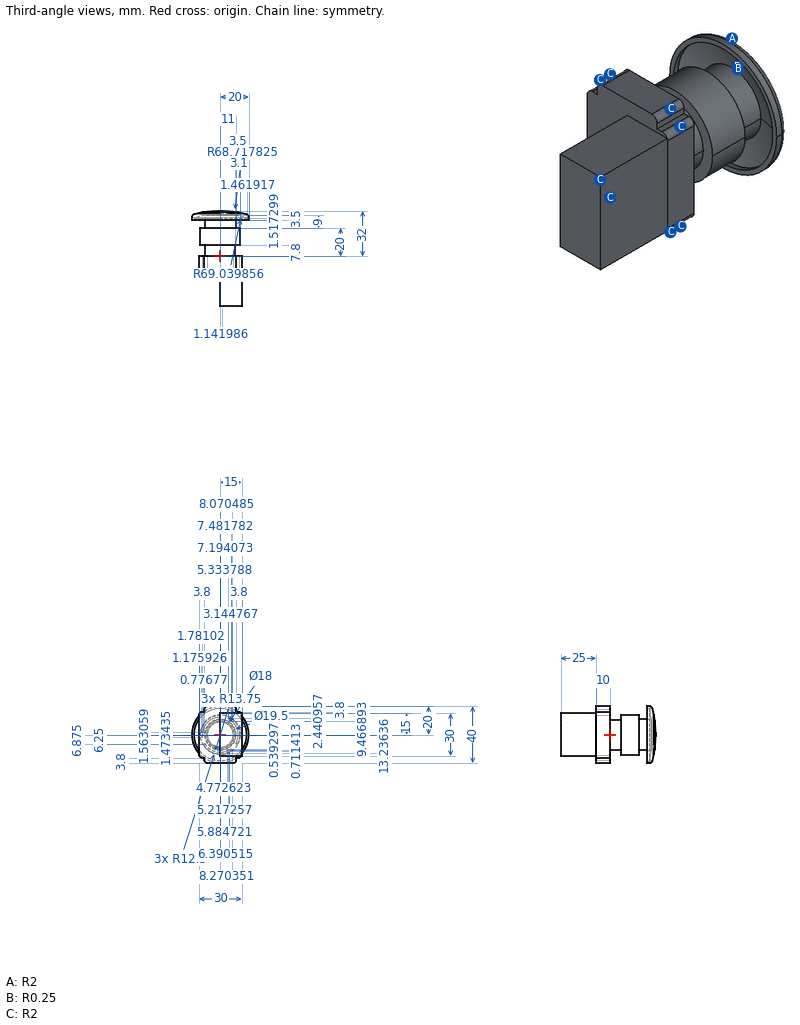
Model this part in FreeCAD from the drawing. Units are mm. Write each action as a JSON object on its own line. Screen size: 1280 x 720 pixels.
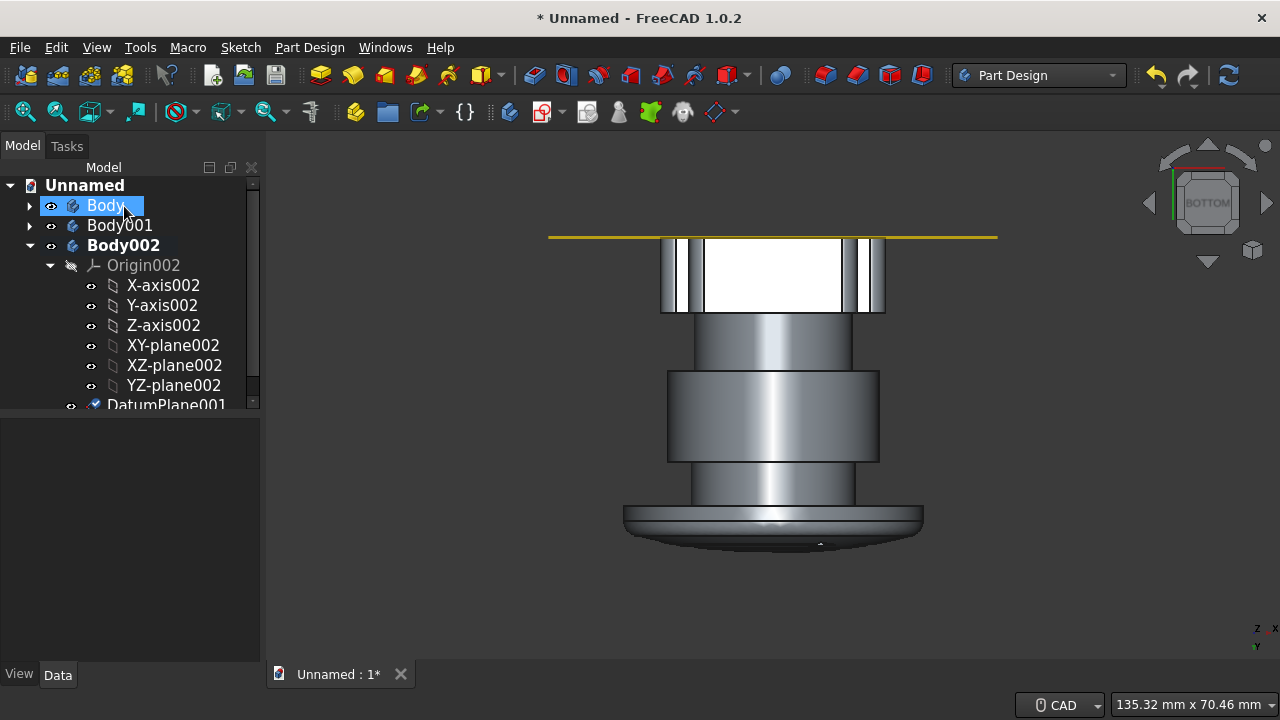
{"action": "left_click", "coordinate": [116, 406]}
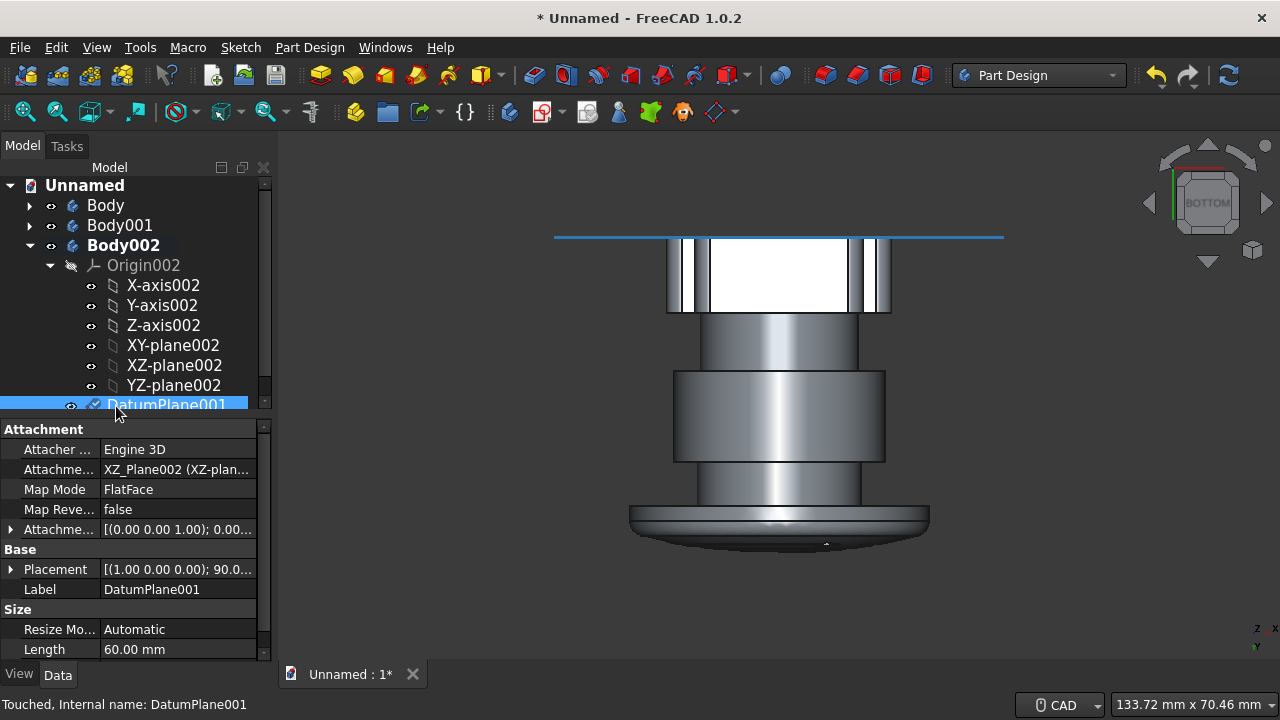
{"action": "left_click", "coordinate": [542, 112]}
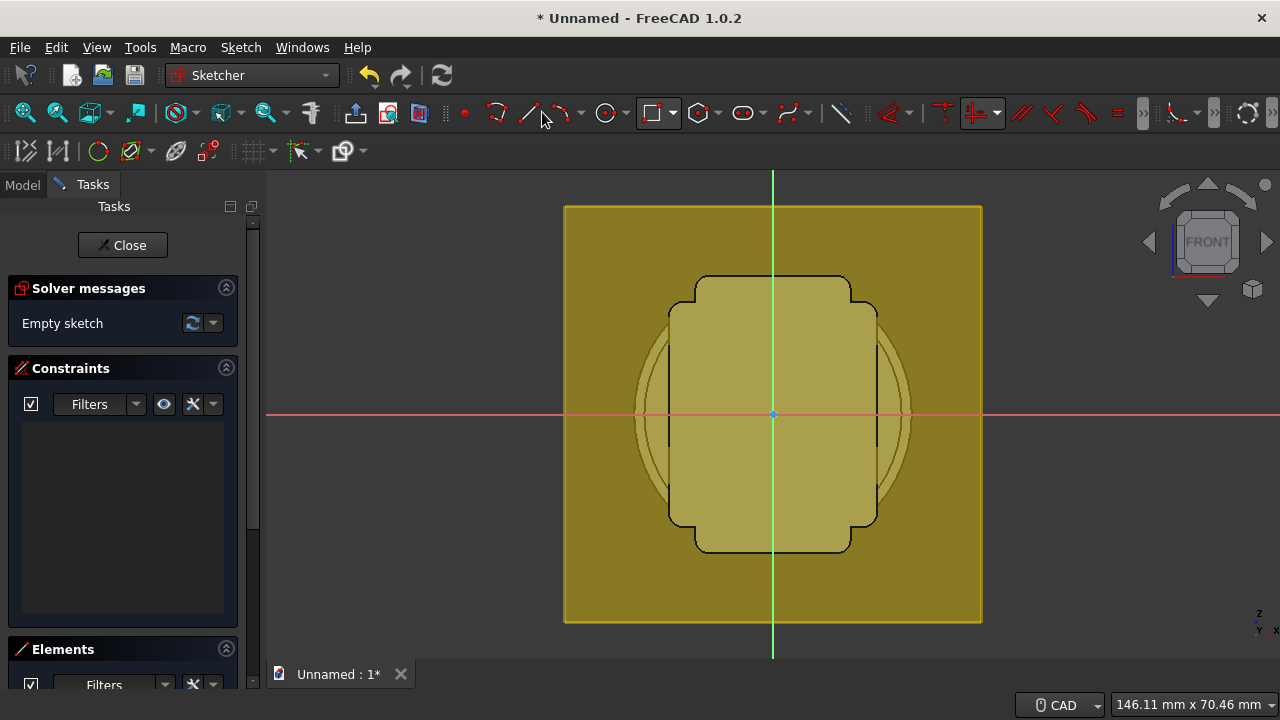
{"action": "scroll", "coordinate": [1070, 414], "scroll_direction": "up", "scroll_amount": 2}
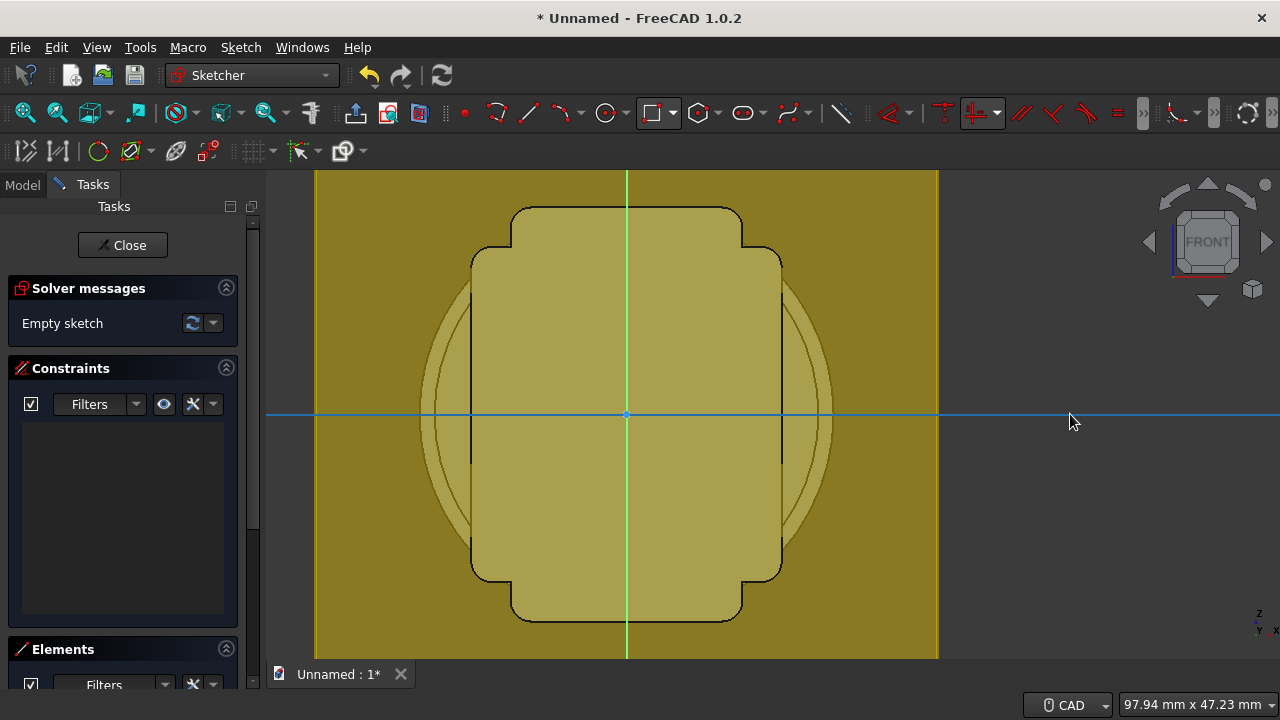
{"action": "left_click", "coordinate": [652, 114]}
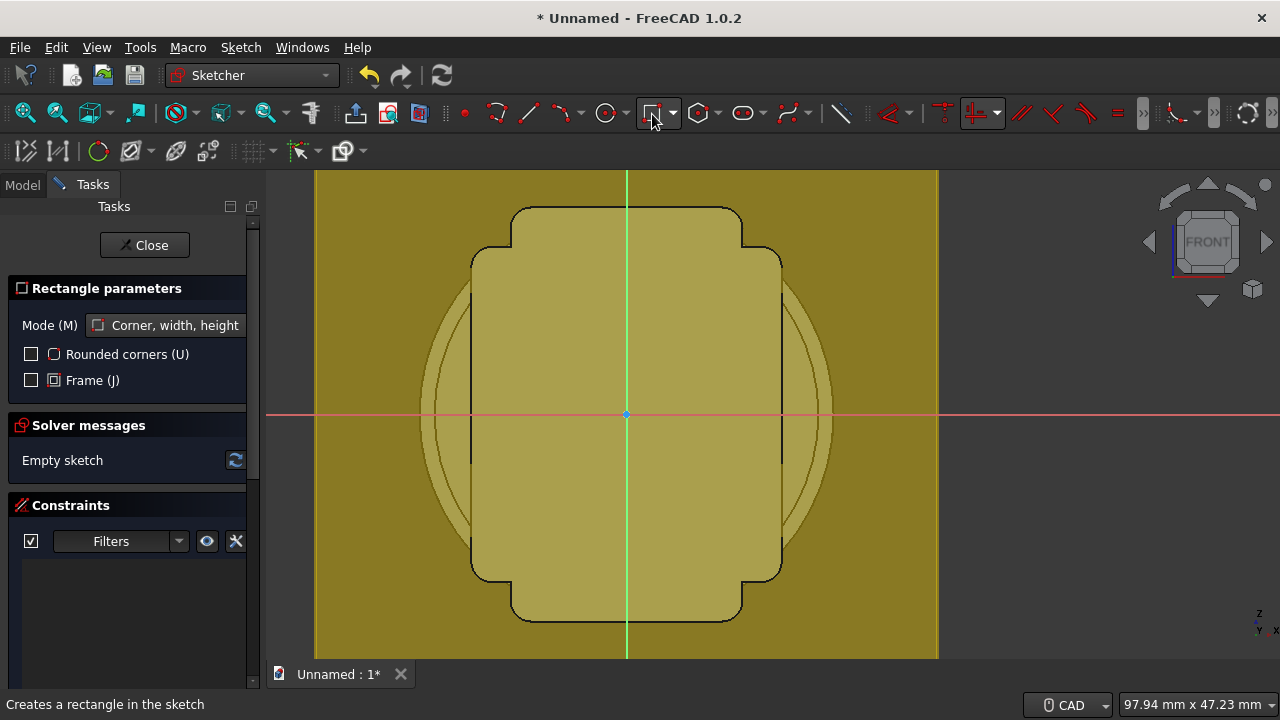
{"action": "left_click", "coordinate": [627, 259]}
{"action": "mouse_move", "coordinate": [782, 570]}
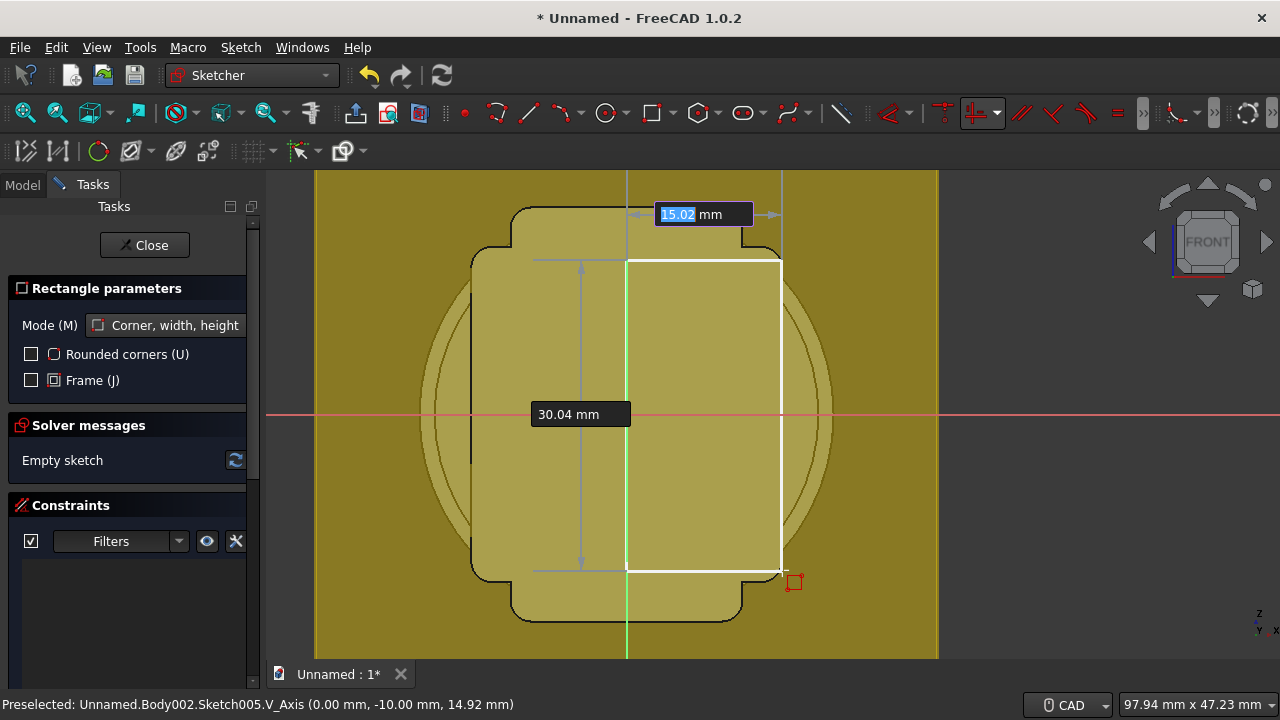
{"action": "type", "text": "15"}
{"action": "key", "text": "Tab"}
{"action": "type", "text": "30"}
{"action": "key", "text": "Return"}
{"action": "key", "text": "Escape"}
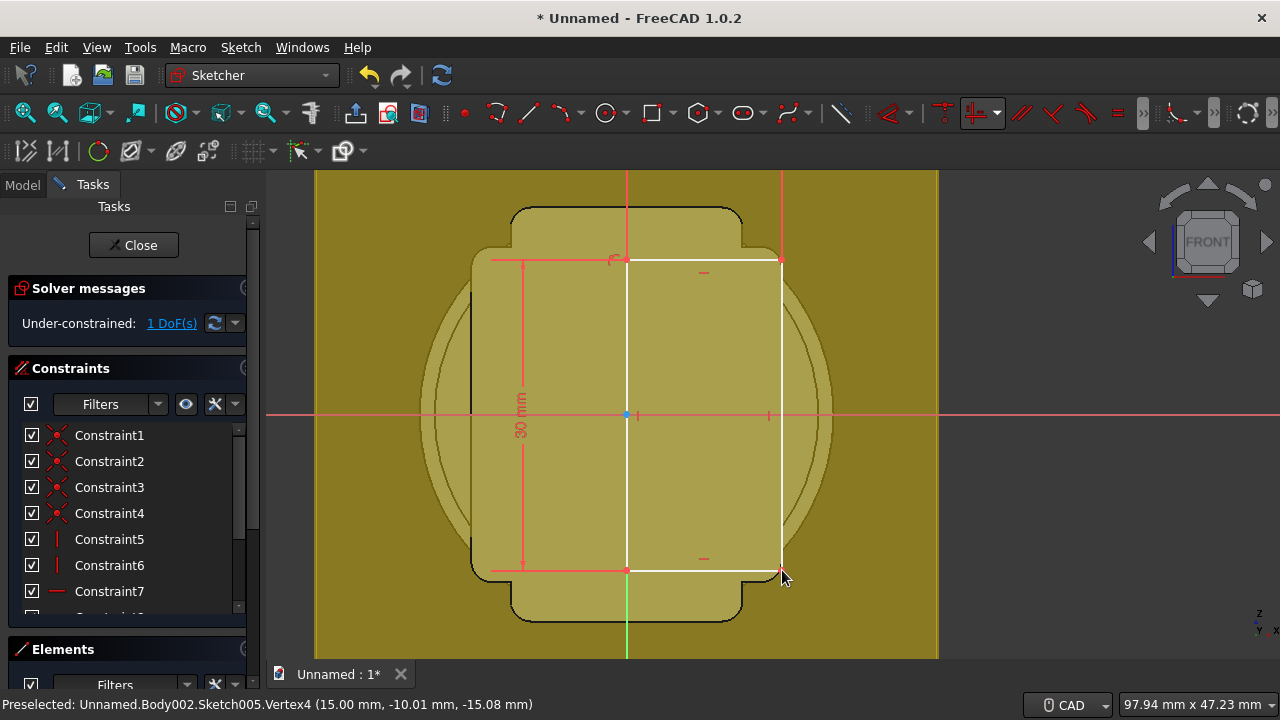
{"action": "left_click", "coordinate": [888, 114]}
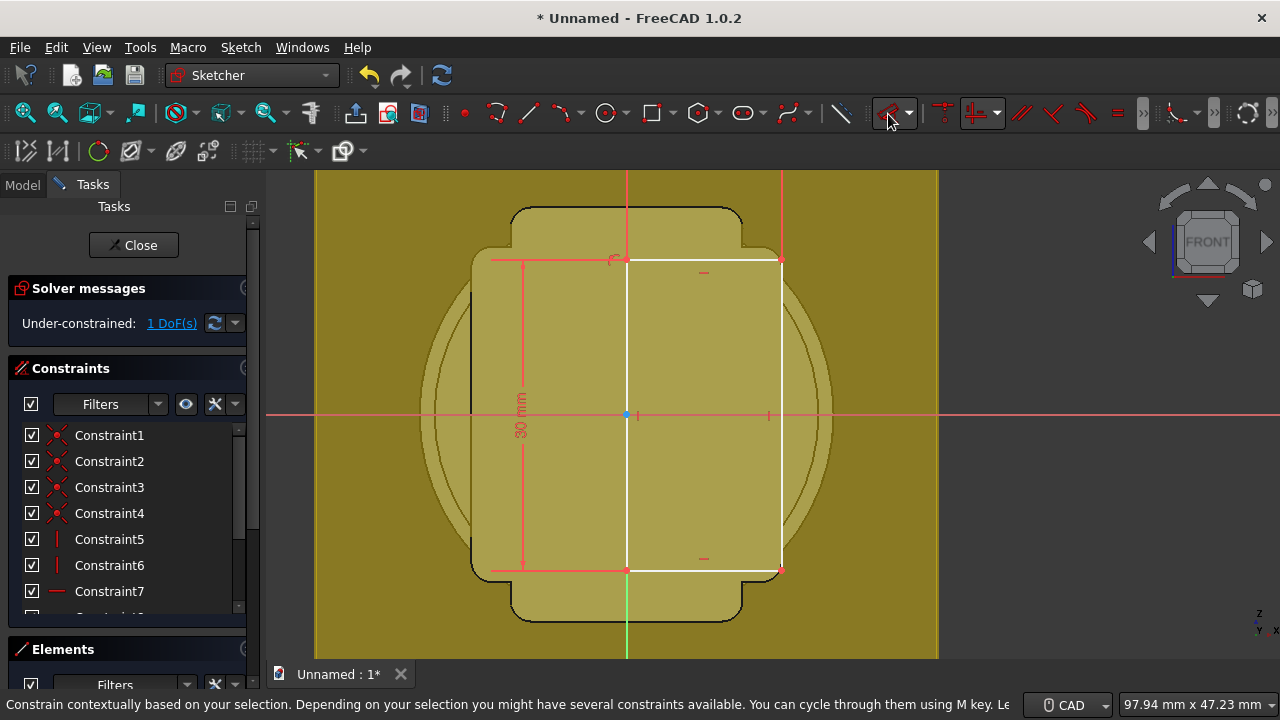
{"action": "left_click", "coordinate": [627, 260]}
{"action": "left_click", "coordinate": [593, 337]}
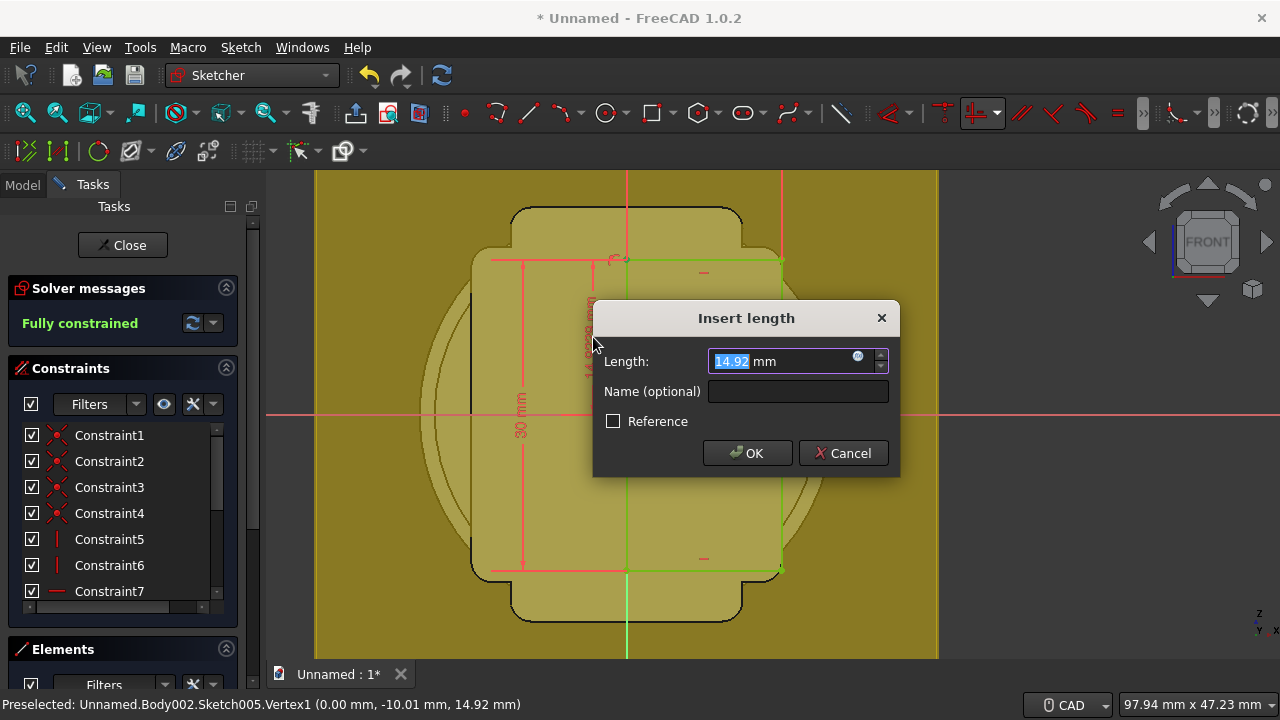
{"action": "type", "text": "15"}
{"action": "key", "text": "Return"}
{"action": "key", "text": "Escape"}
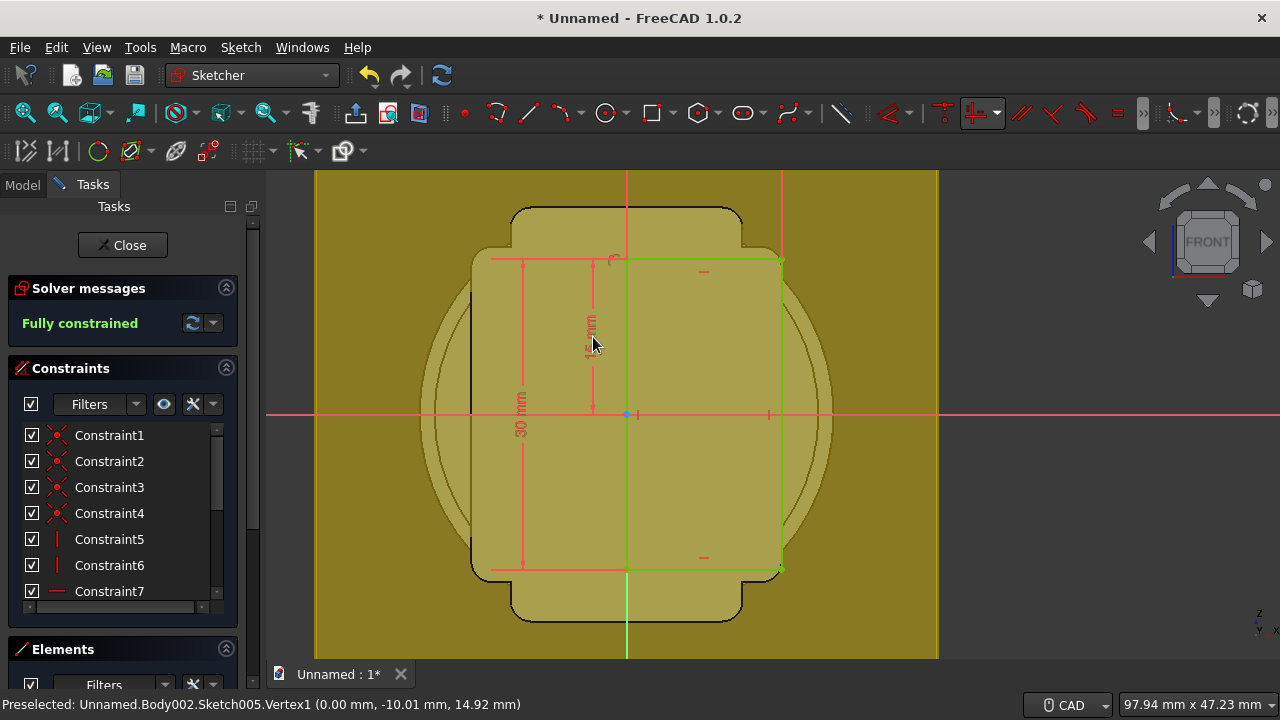
{"action": "left_click", "coordinate": [123, 245]}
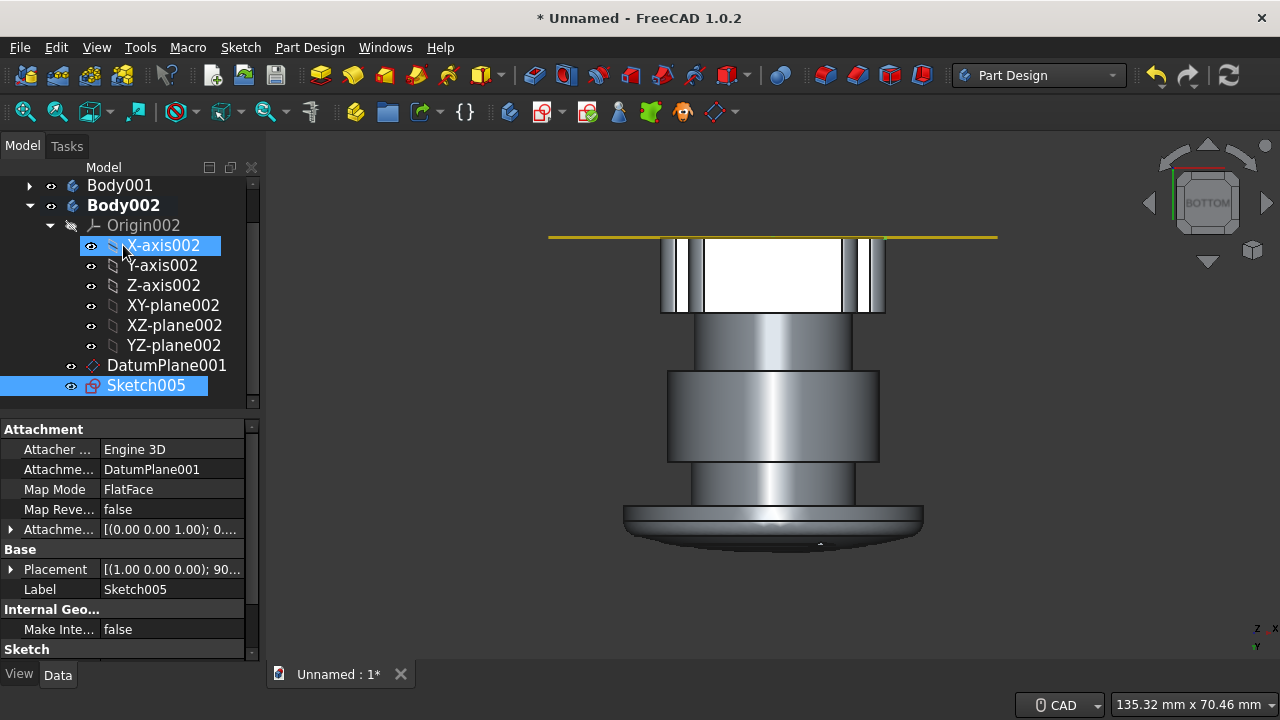
{"action": "left_click", "coordinate": [322, 76]}